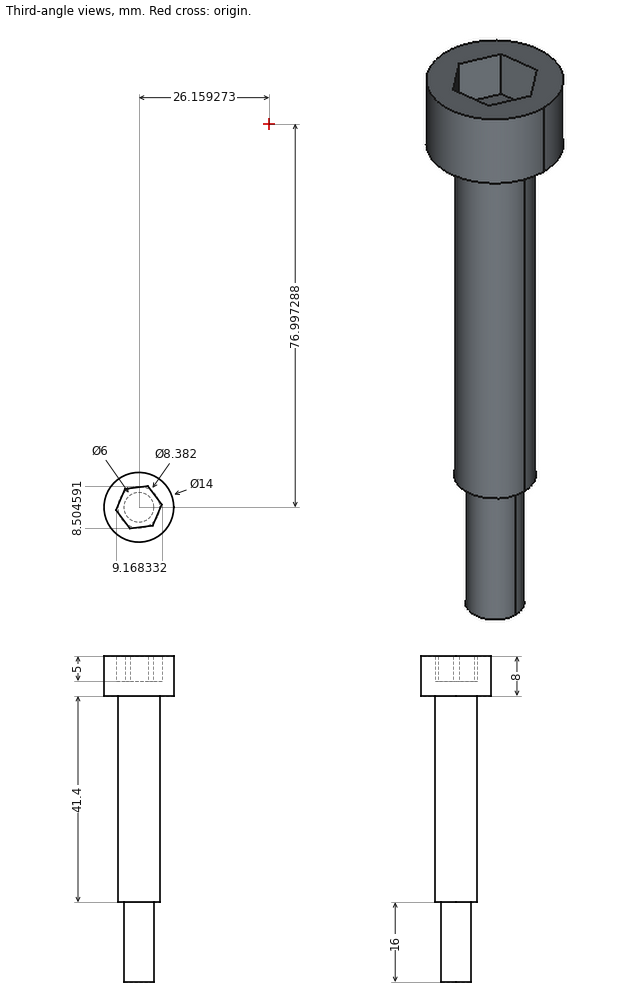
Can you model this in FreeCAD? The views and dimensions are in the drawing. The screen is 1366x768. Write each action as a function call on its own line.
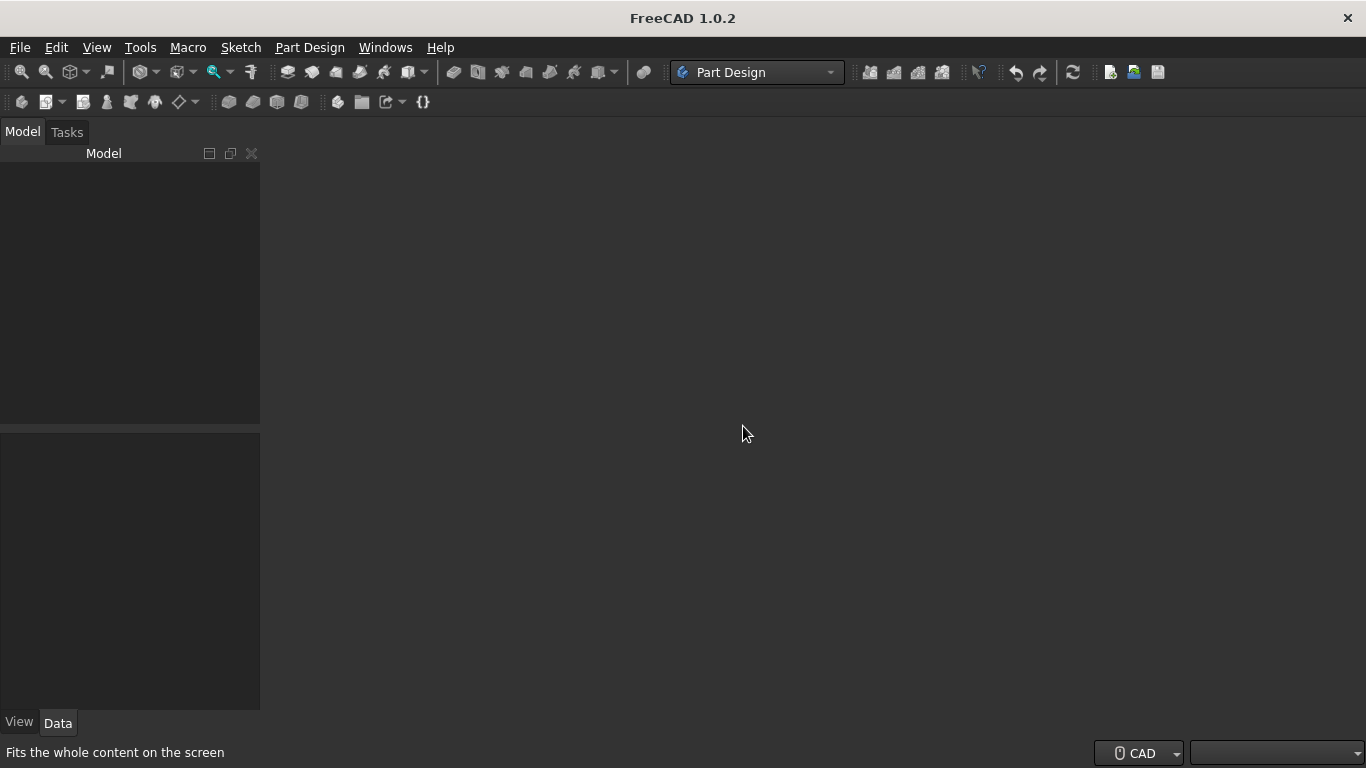
key(ctrl+n)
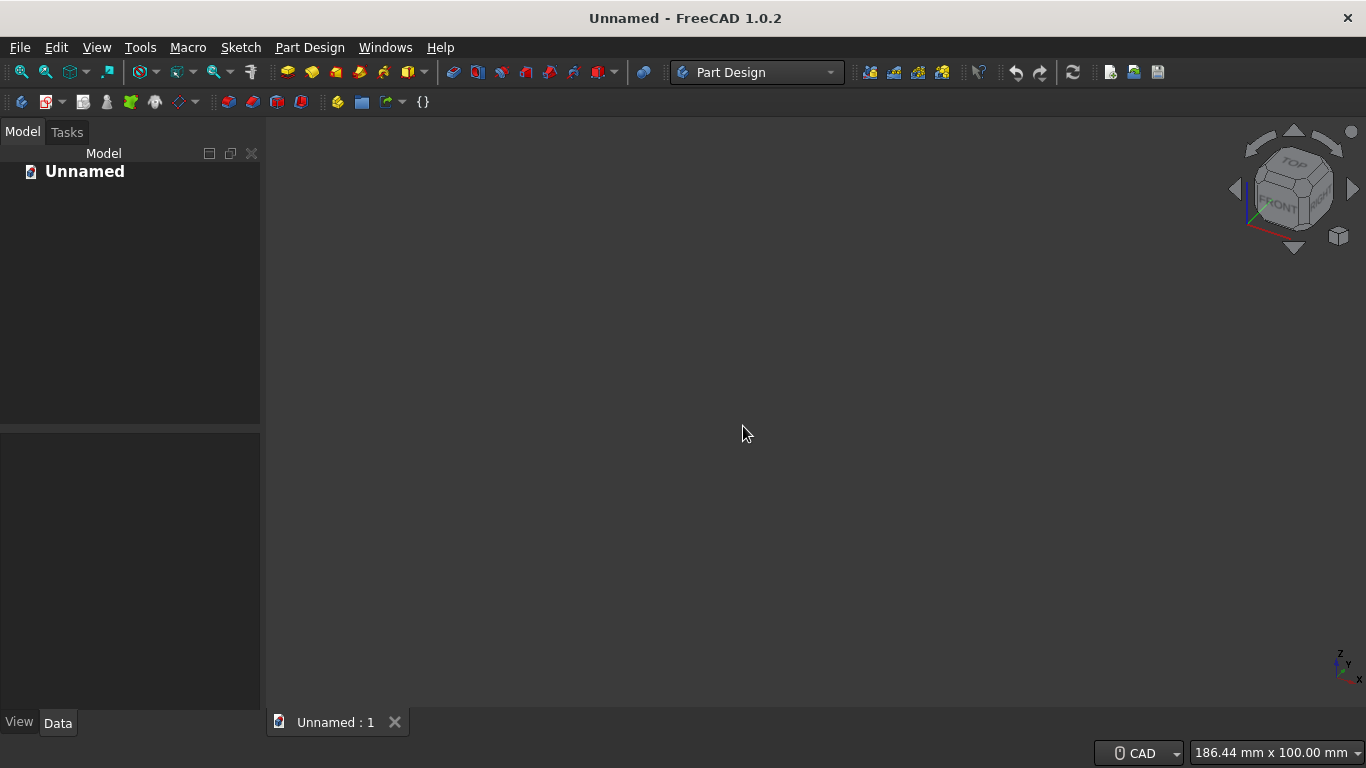
click(46, 102)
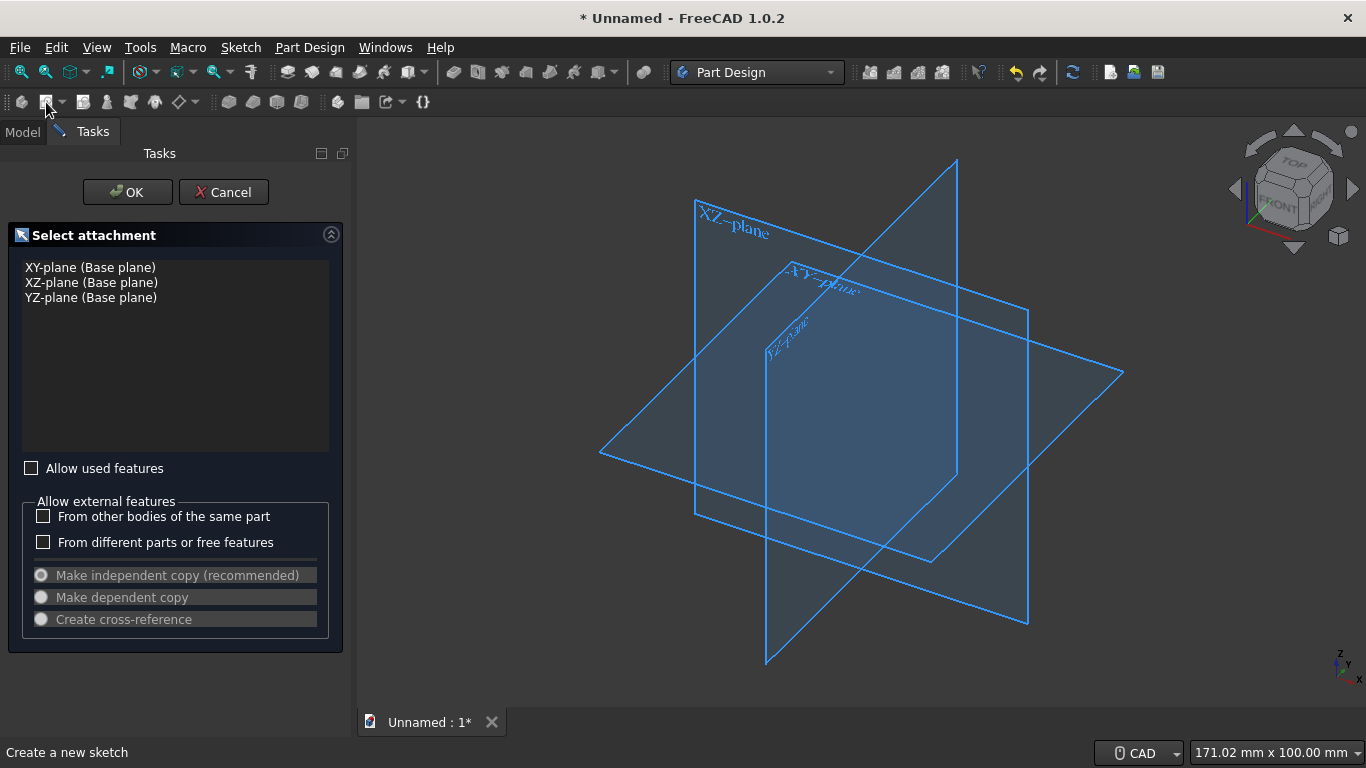
click(82, 268)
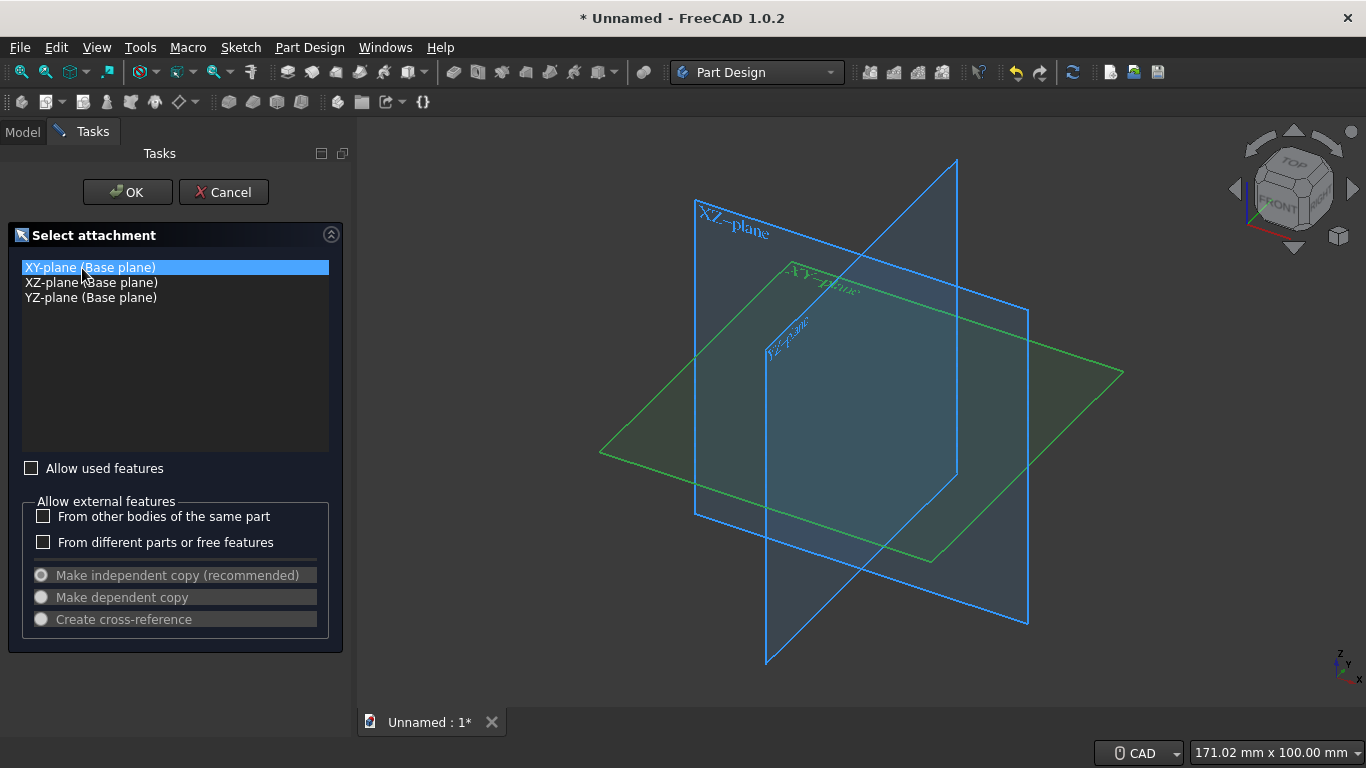
click(128, 192)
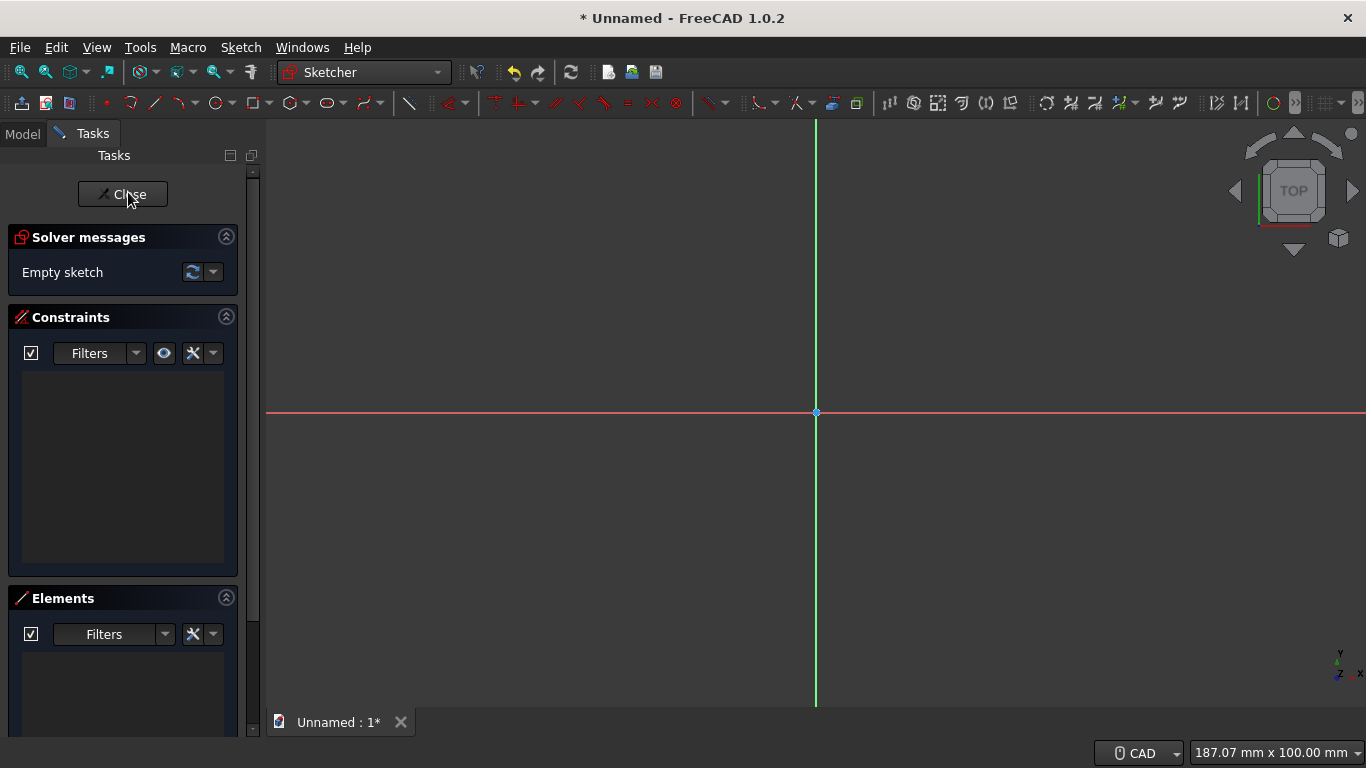
scroll(748, 413, down, 5)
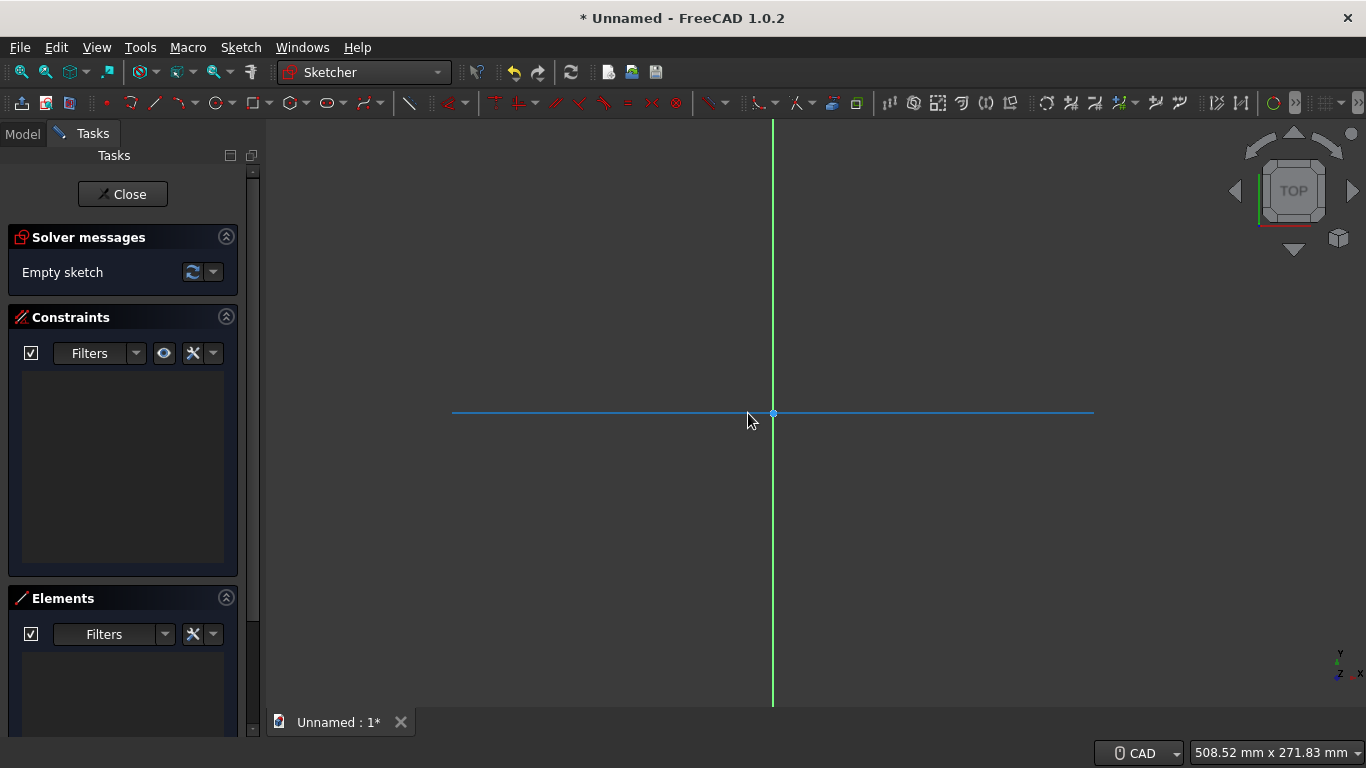
scroll(714, 593, up, 13)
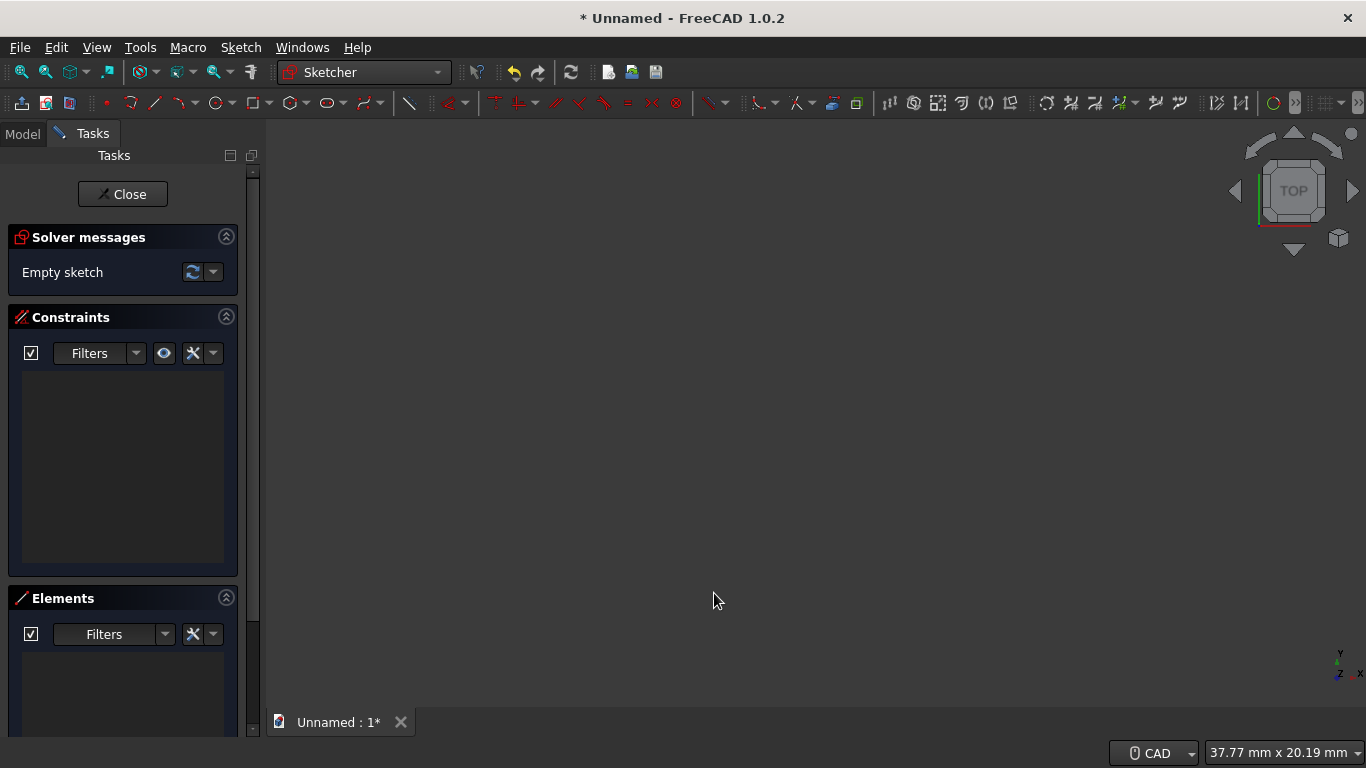
click(216, 104)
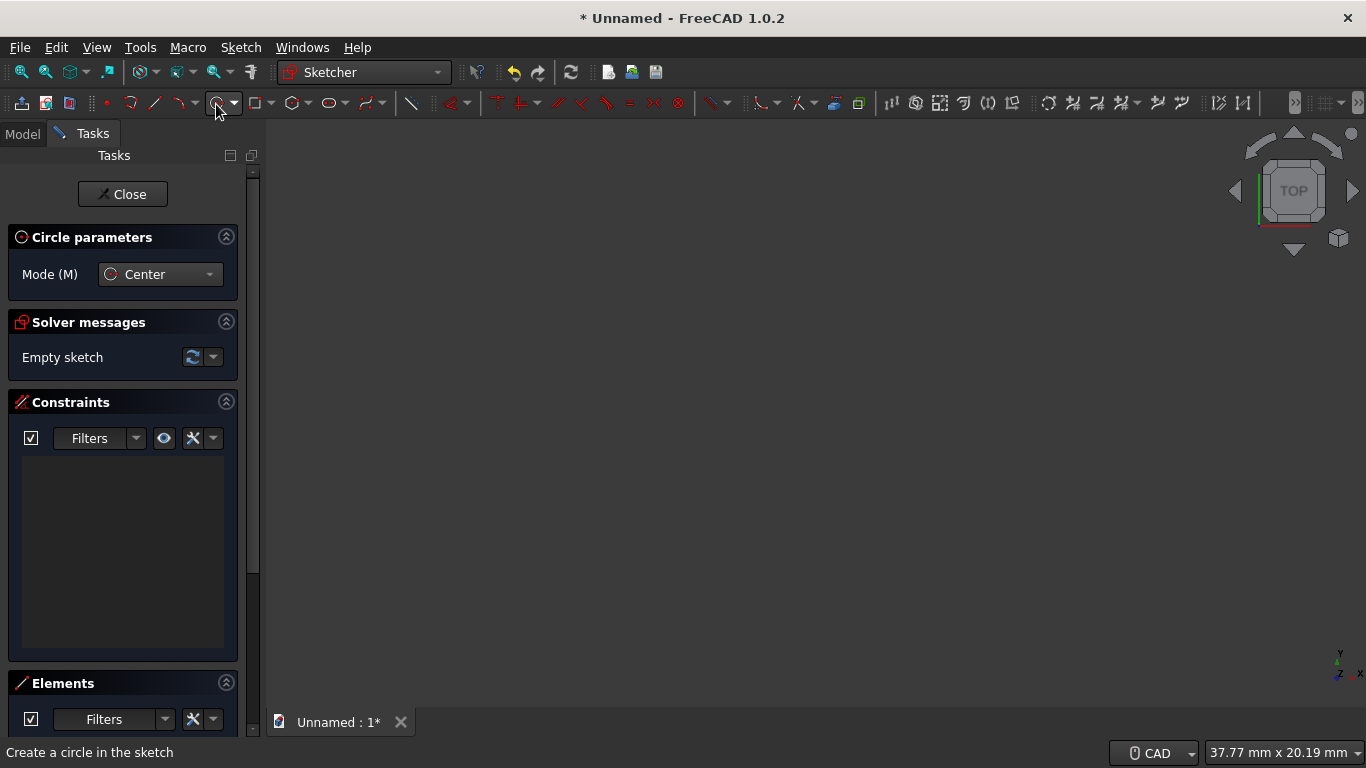
click(745, 406)
move(890, 262)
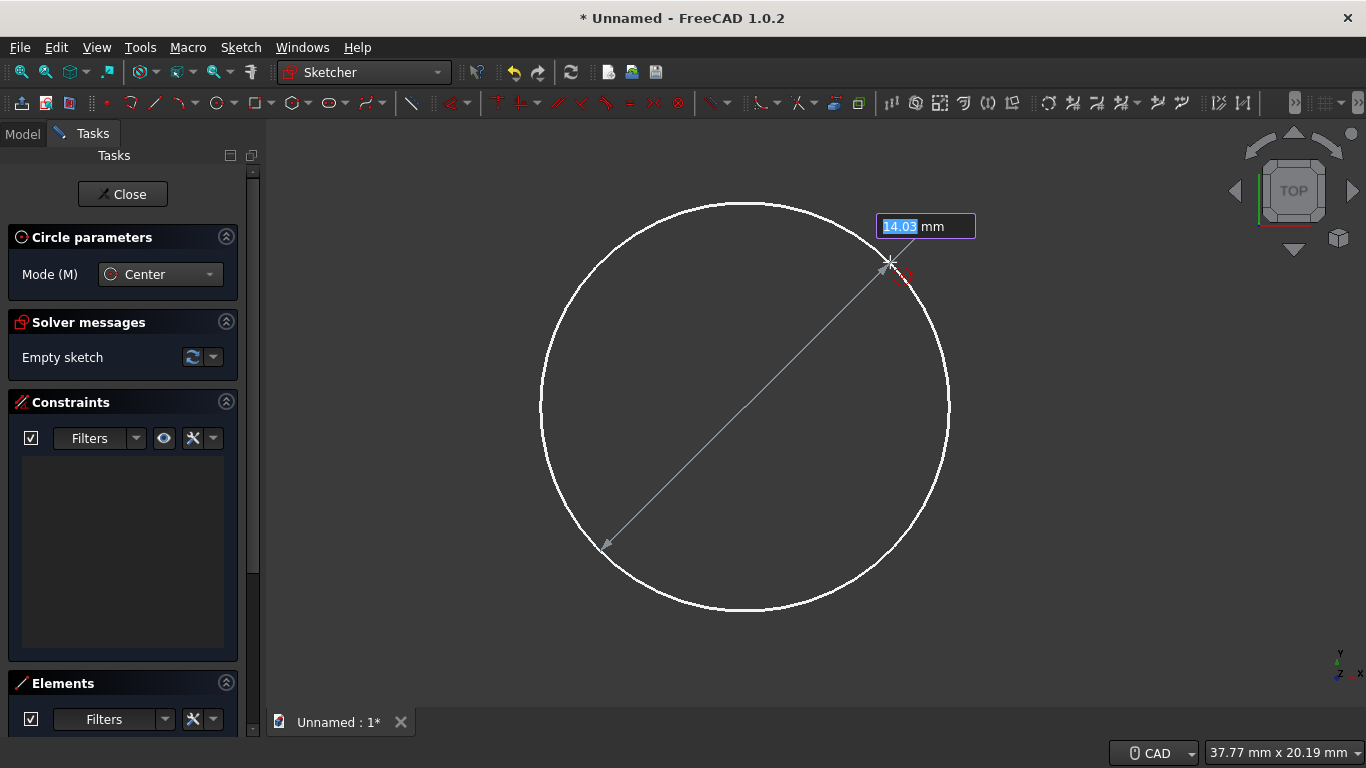
text(14)
key(Return)
key(Escape)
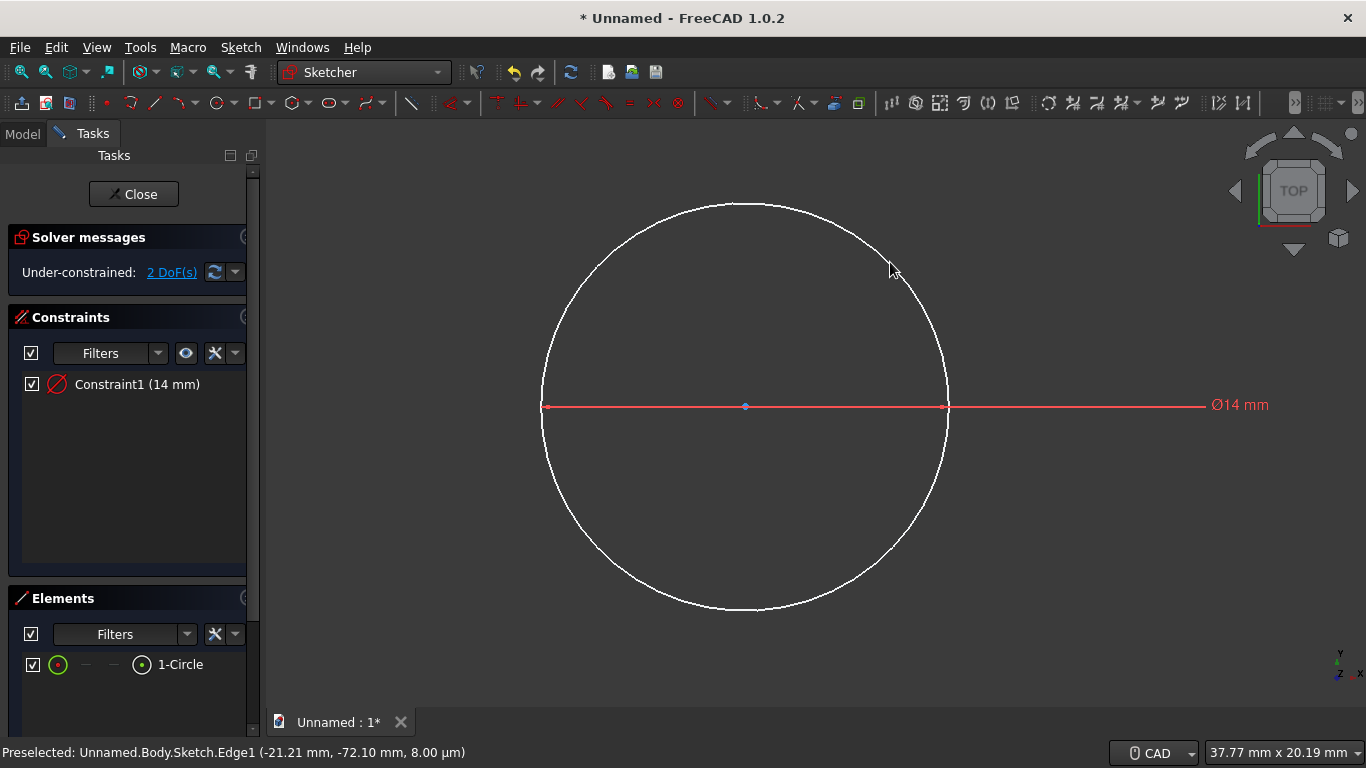
key(d)